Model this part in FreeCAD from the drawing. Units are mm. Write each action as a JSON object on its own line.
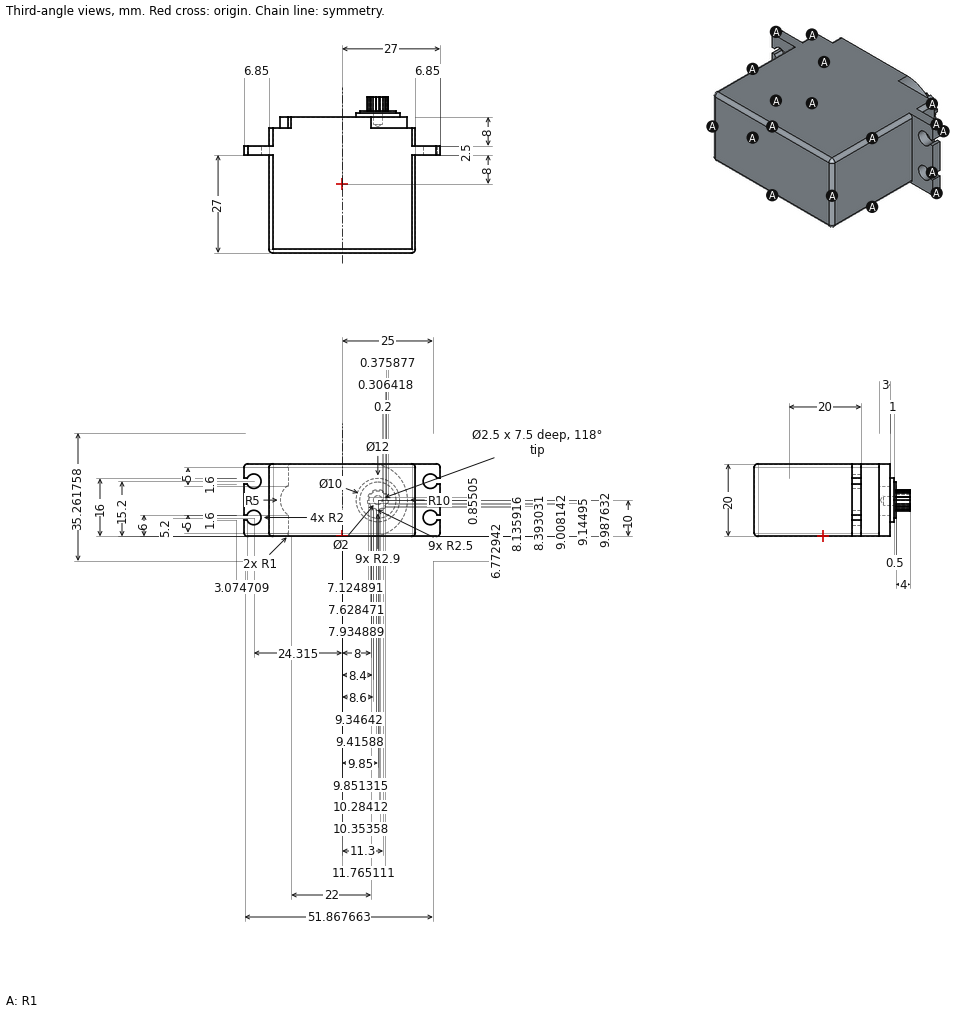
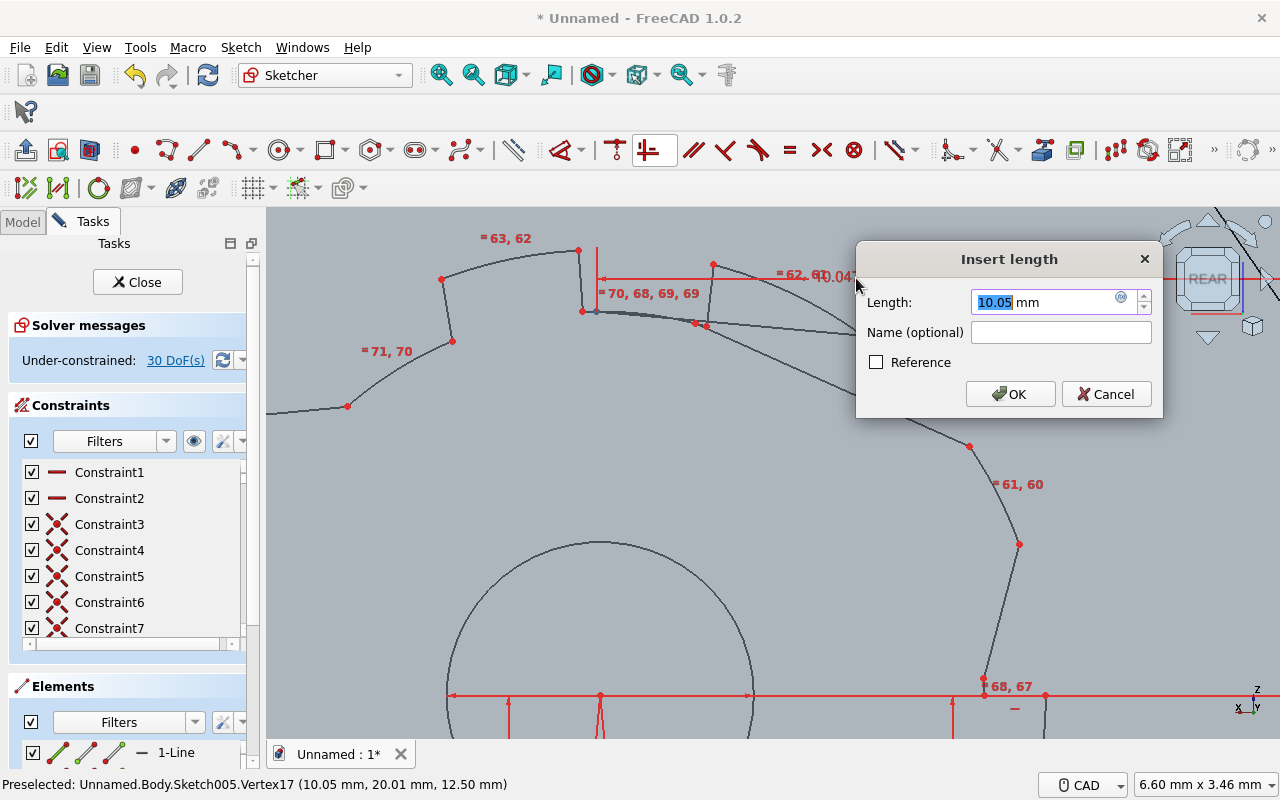
{"action": "type", "text": "8.6"}
{"action": "key", "text": "Return"}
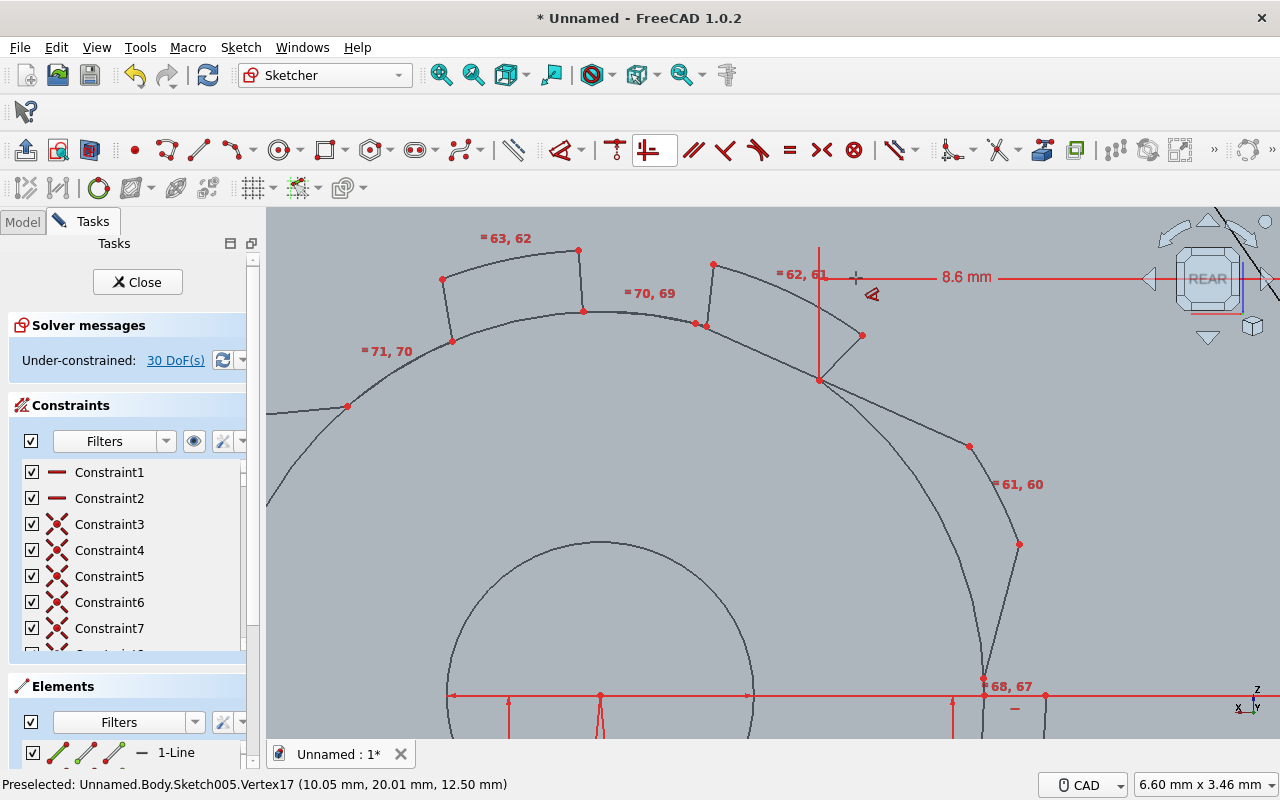
{"action": "scroll", "coordinate": [614, 320], "scroll_direction": "down", "scroll_amount": 9}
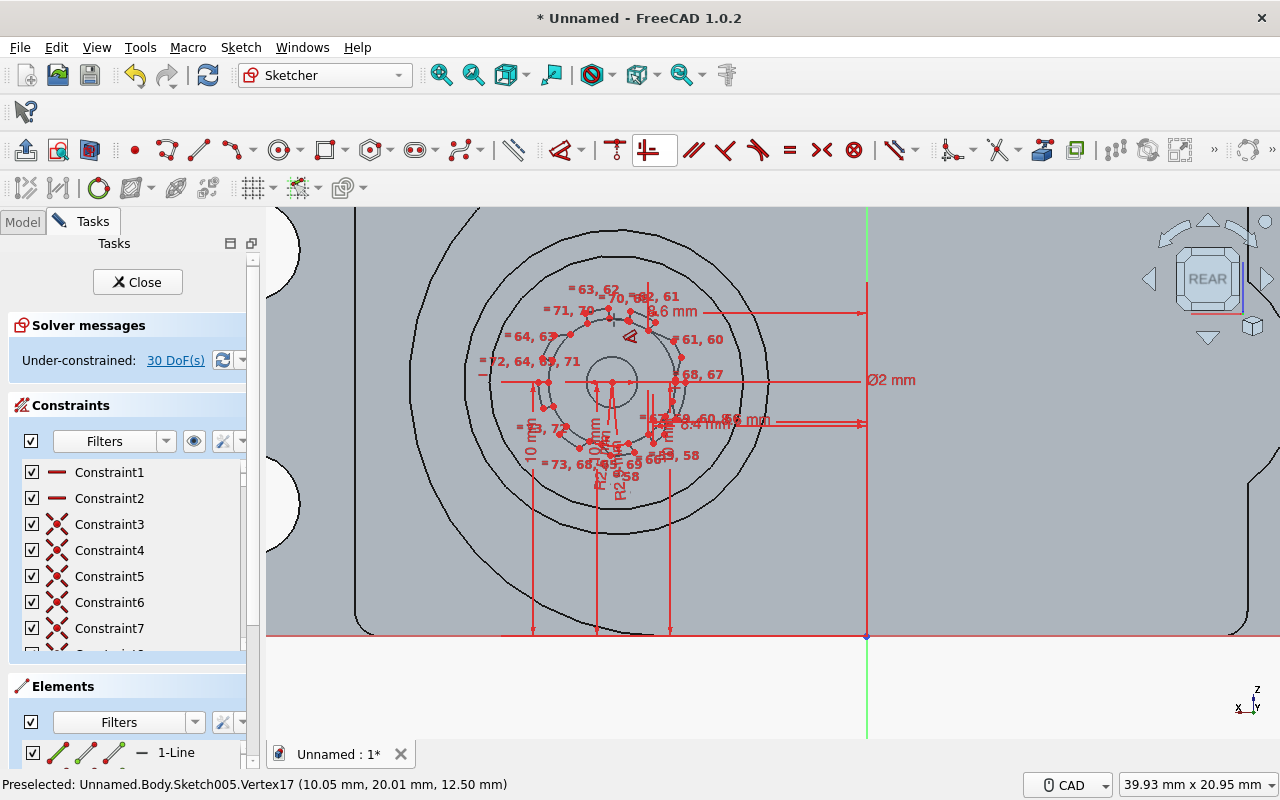
{"action": "left_click", "coordinate": [655, 323]}
{"action": "left_click", "coordinate": [761, 670]}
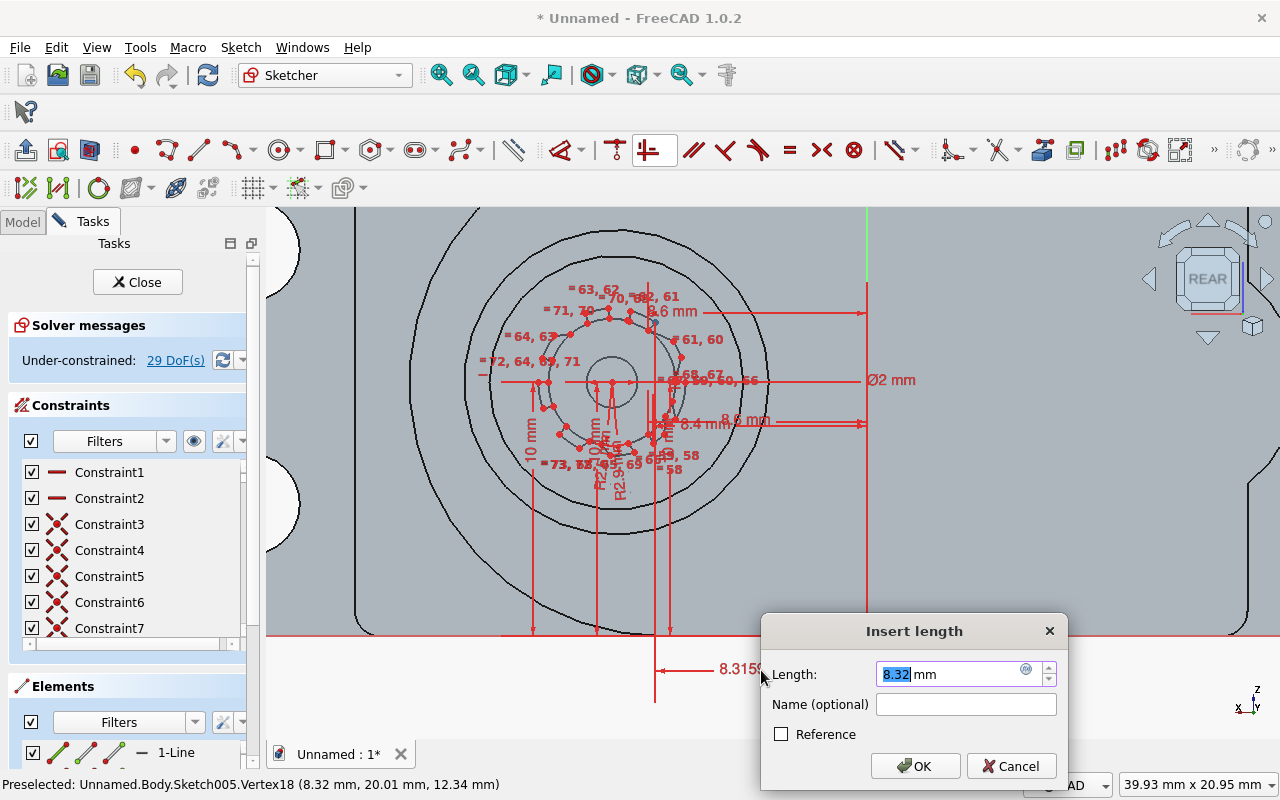
{"action": "type", "text": "8.4"}
{"action": "key", "text": "Return"}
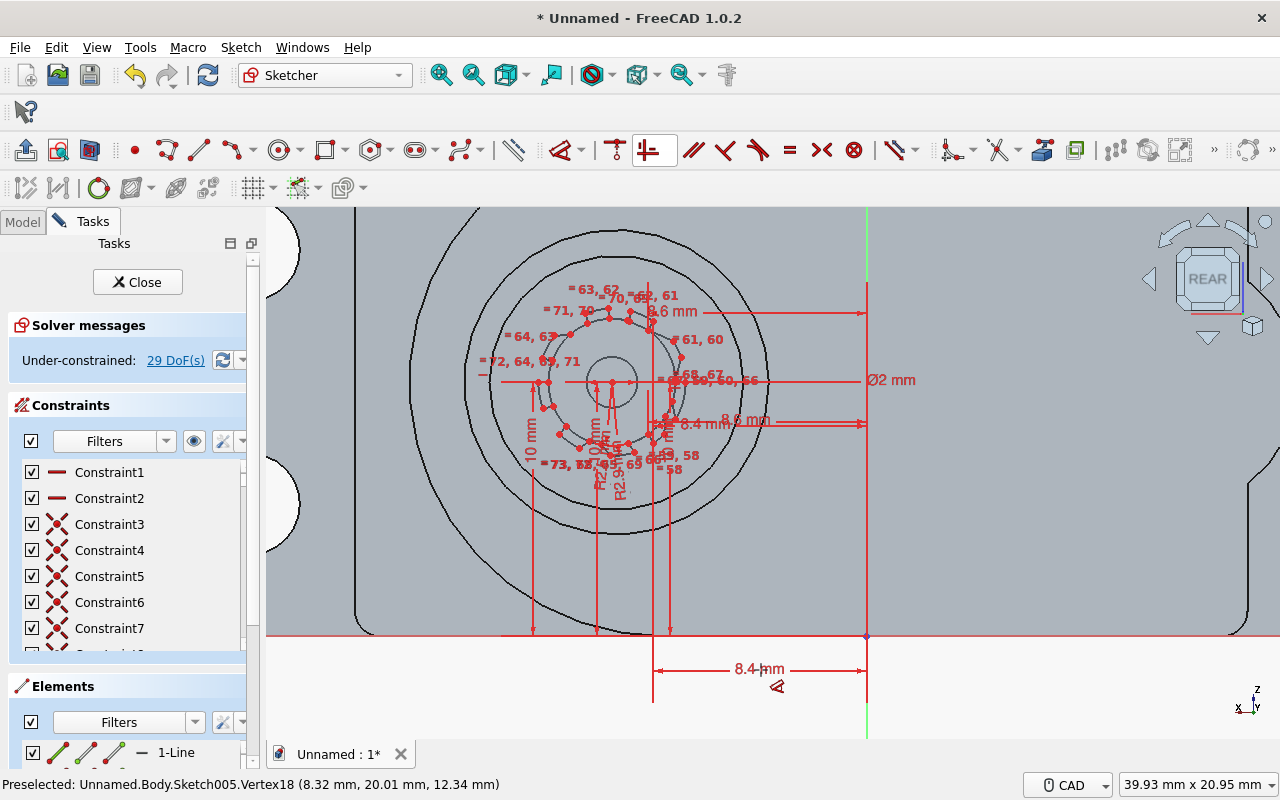
{"action": "scroll", "coordinate": [587, 319], "scroll_direction": "up", "scroll_amount": 11}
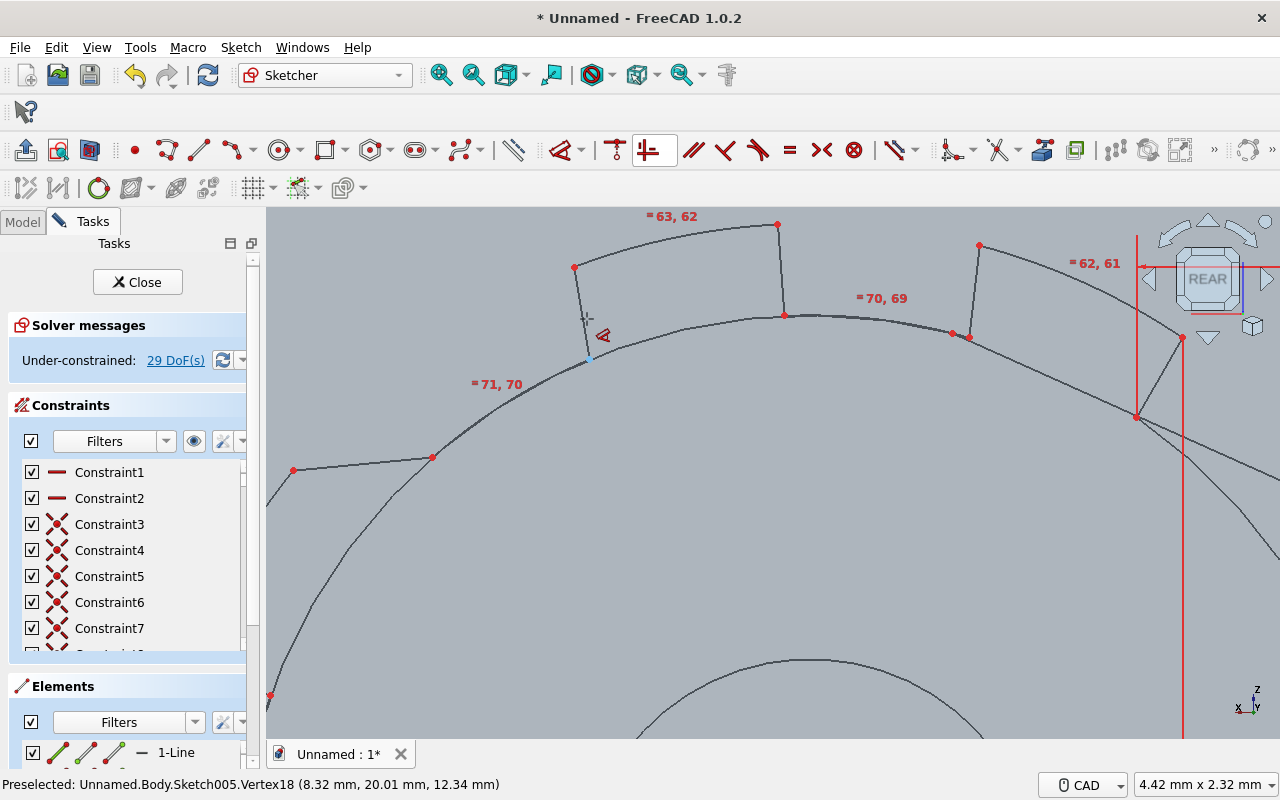
{"action": "left_click", "coordinate": [582, 313]}
{"action": "left_click", "coordinate": [582, 394]}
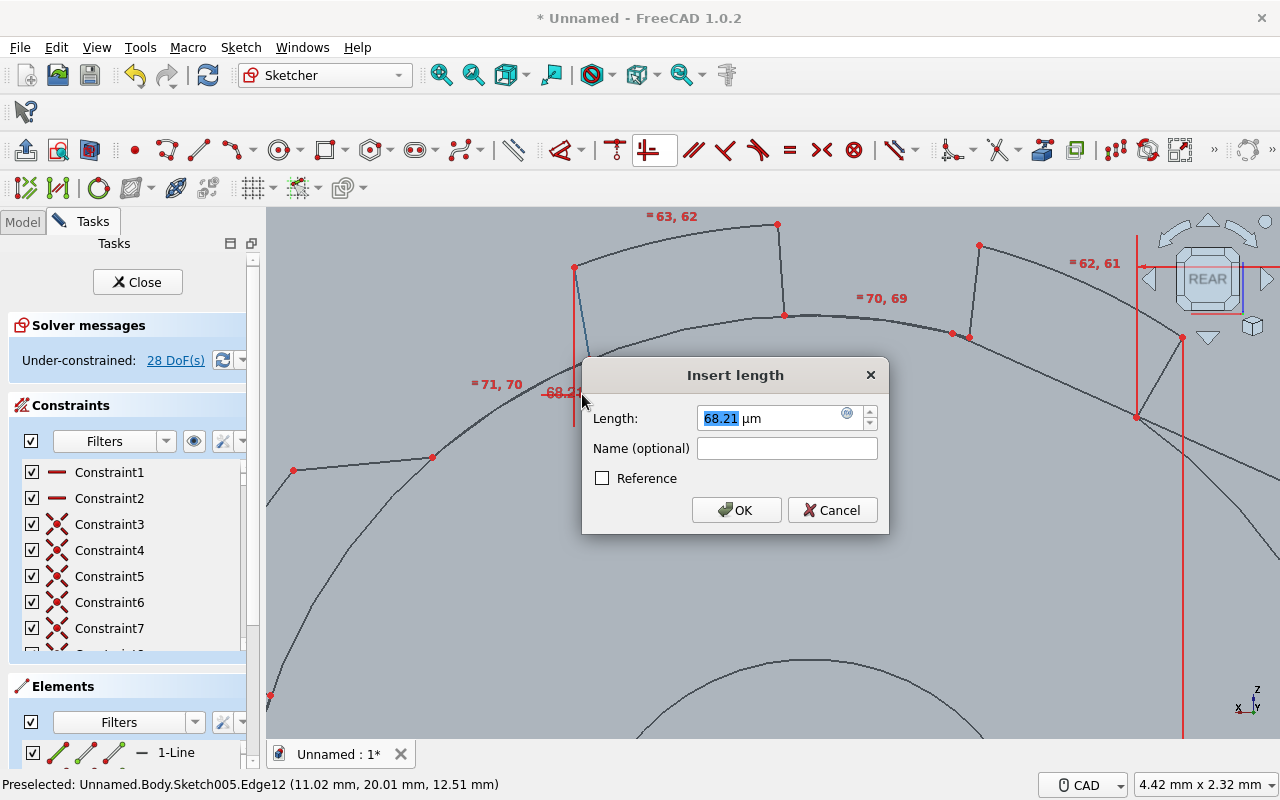
{"action": "key", "text": "ctrl+a"}
{"action": "type", "text": "0.2 mm"}
{"action": "key", "text": "Return"}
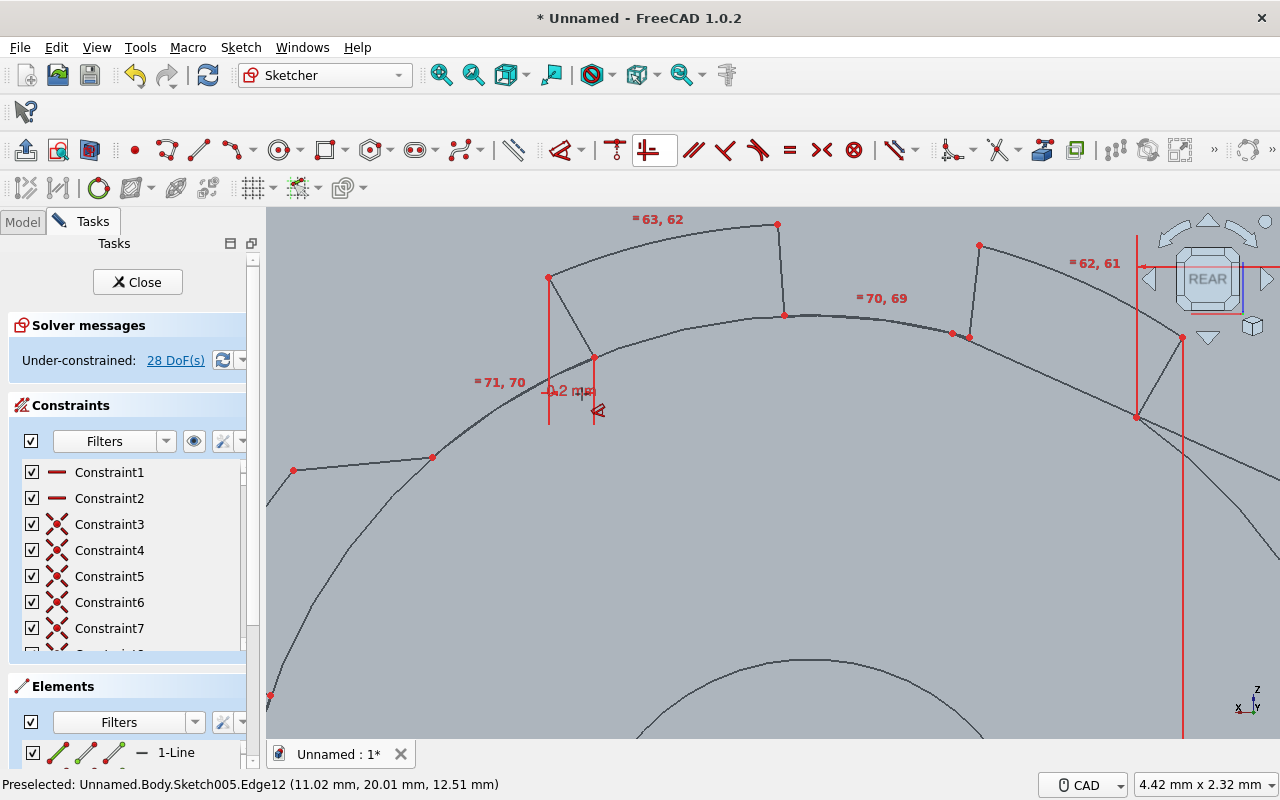
{"action": "scroll", "coordinate": [587, 319], "scroll_direction": "down", "scroll_amount": 11}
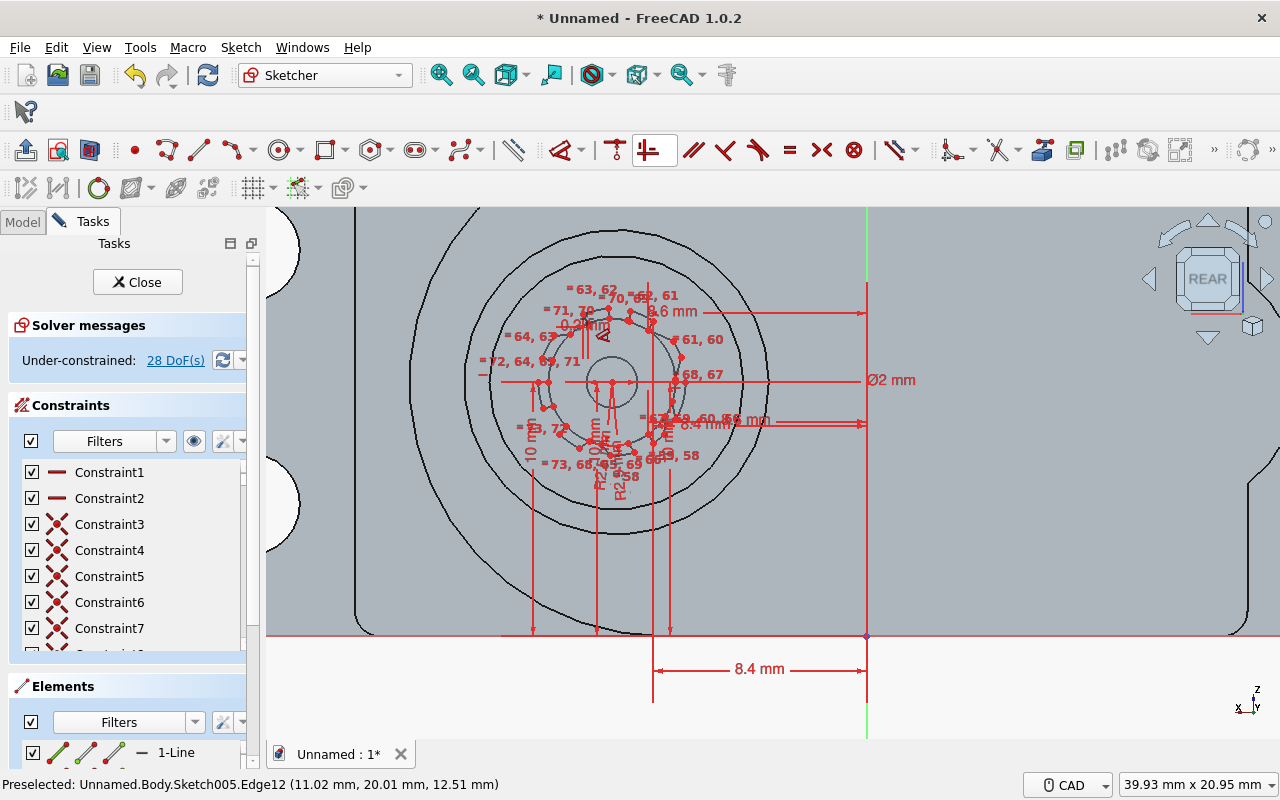
{"action": "scroll", "coordinate": [582, 446], "scroll_direction": "up", "scroll_amount": 11}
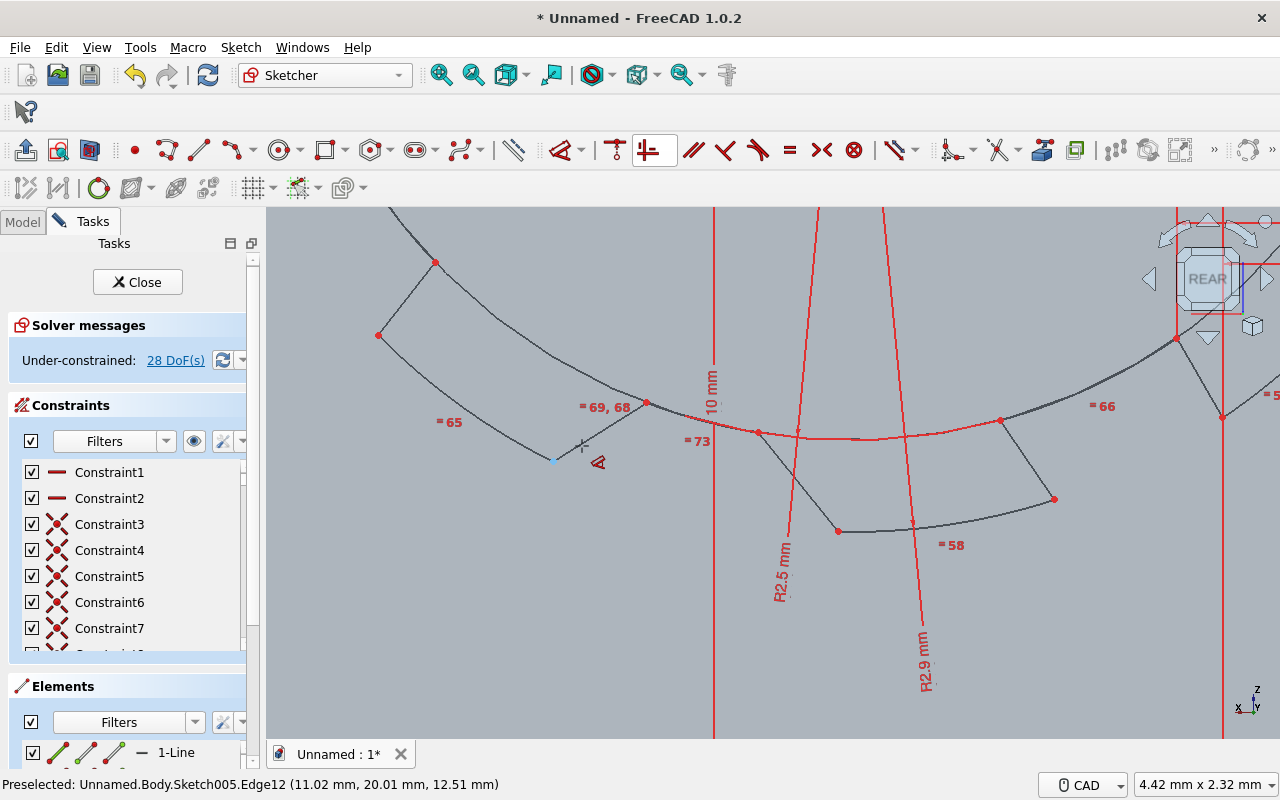
{"action": "left_click", "coordinate": [581, 444]}
{"action": "left_click", "coordinate": [622, 369]}